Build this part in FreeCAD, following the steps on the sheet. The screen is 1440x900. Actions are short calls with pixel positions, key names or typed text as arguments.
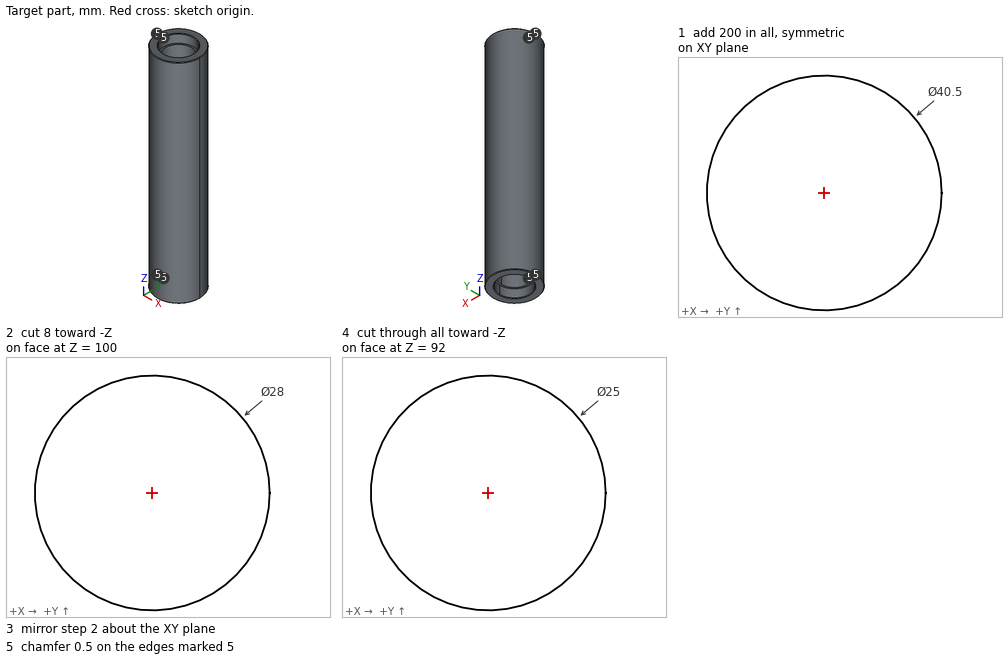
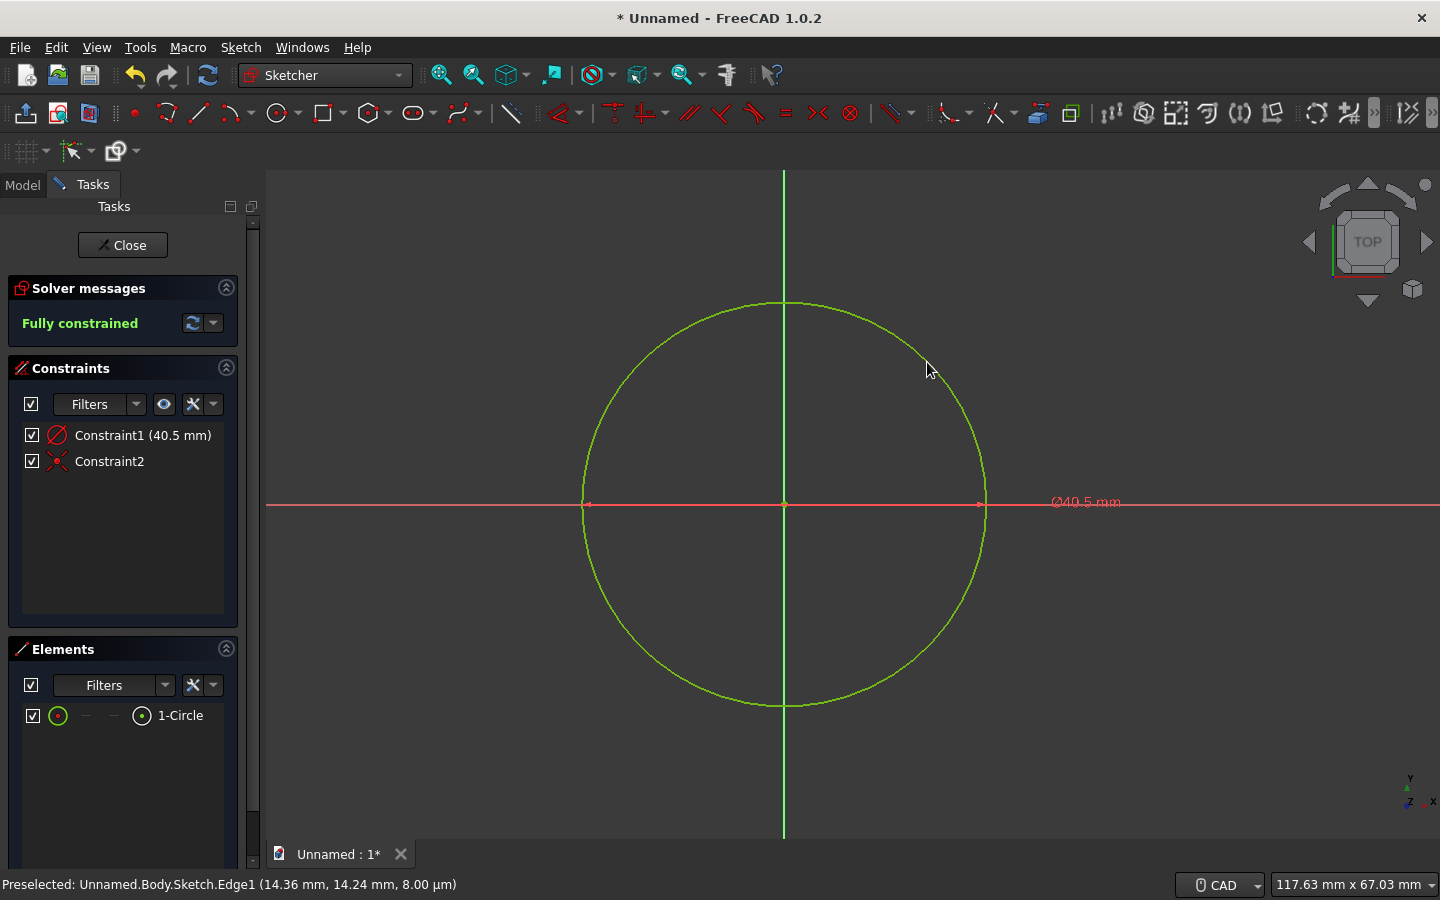
click(123, 245)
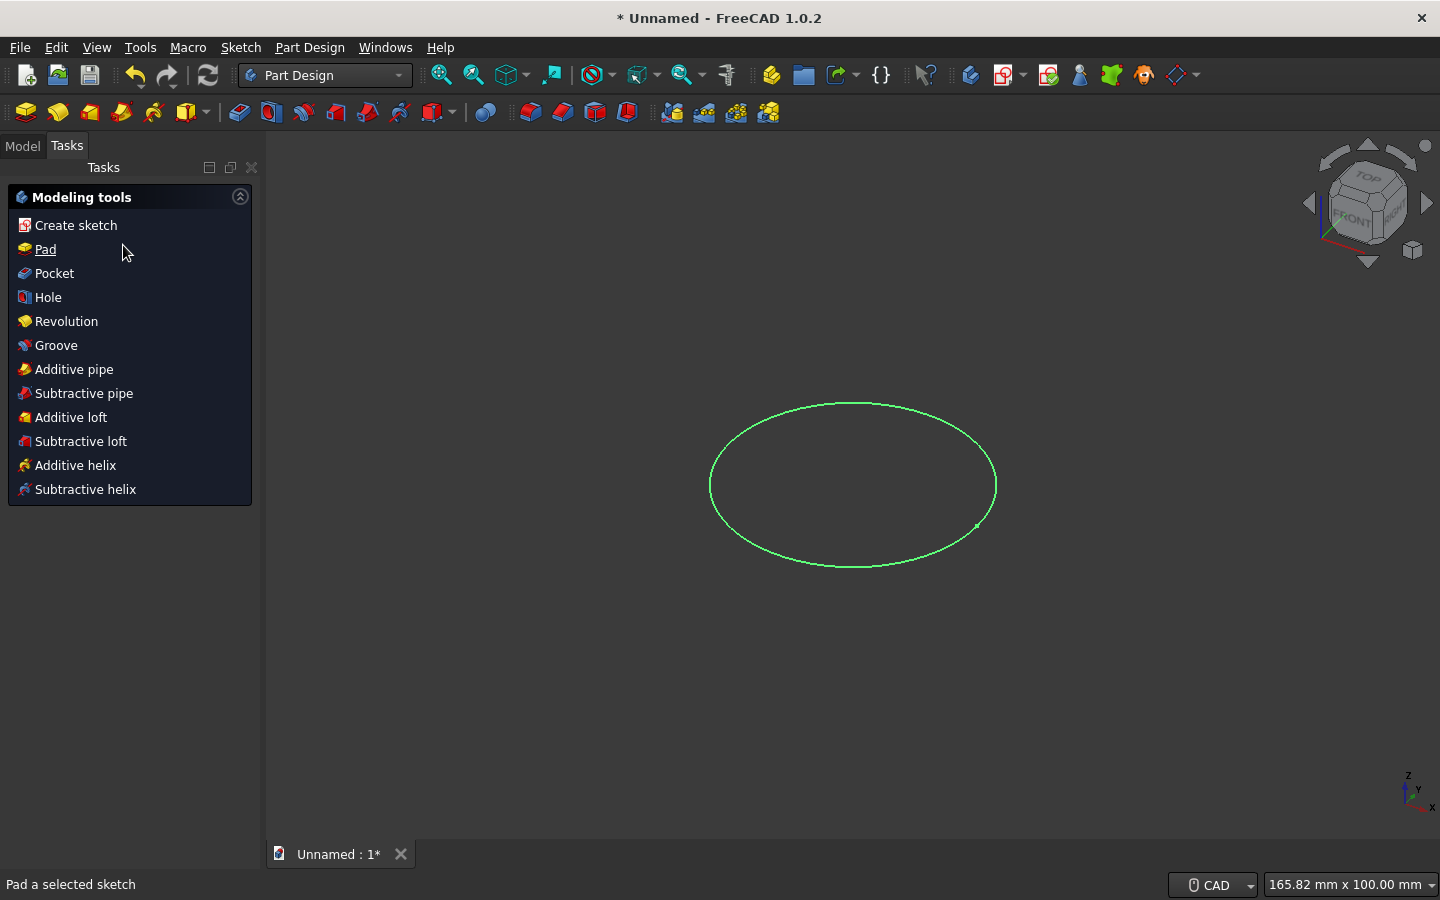
click(26, 112)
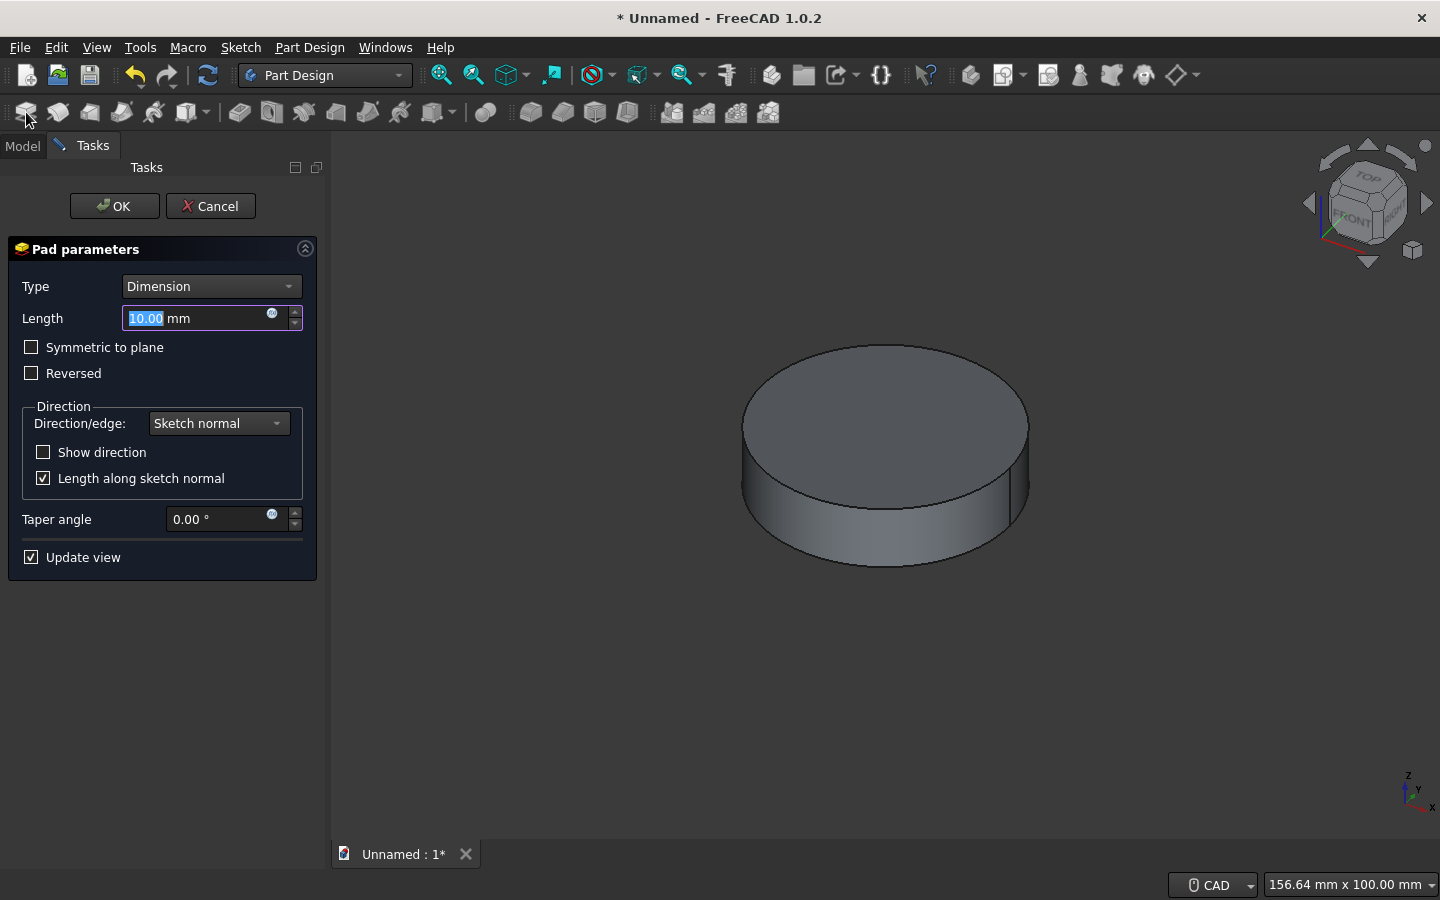
text(200)
key(Tab)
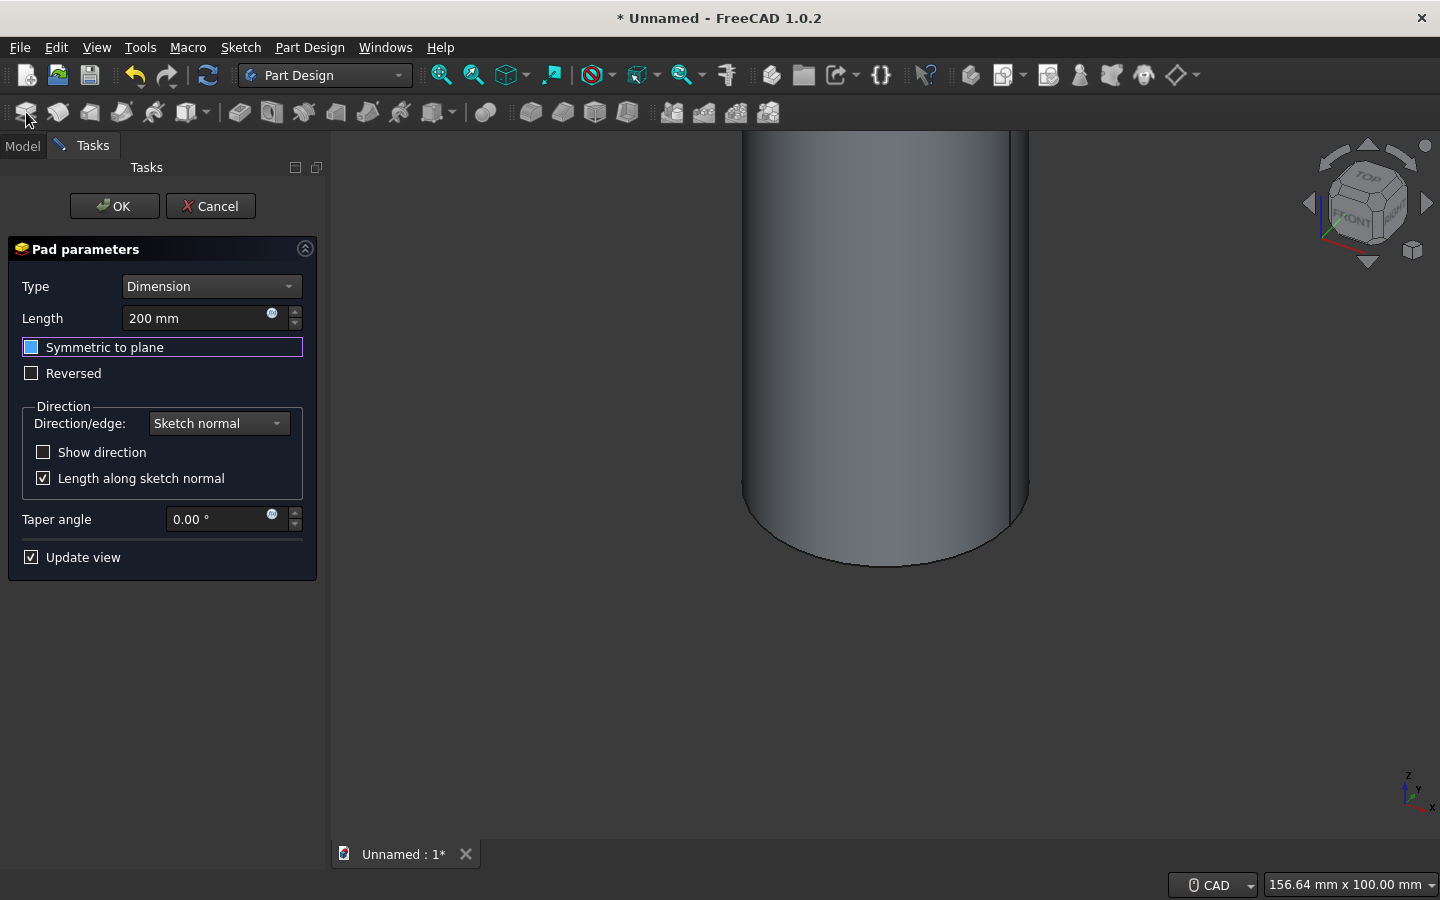
click(30, 347)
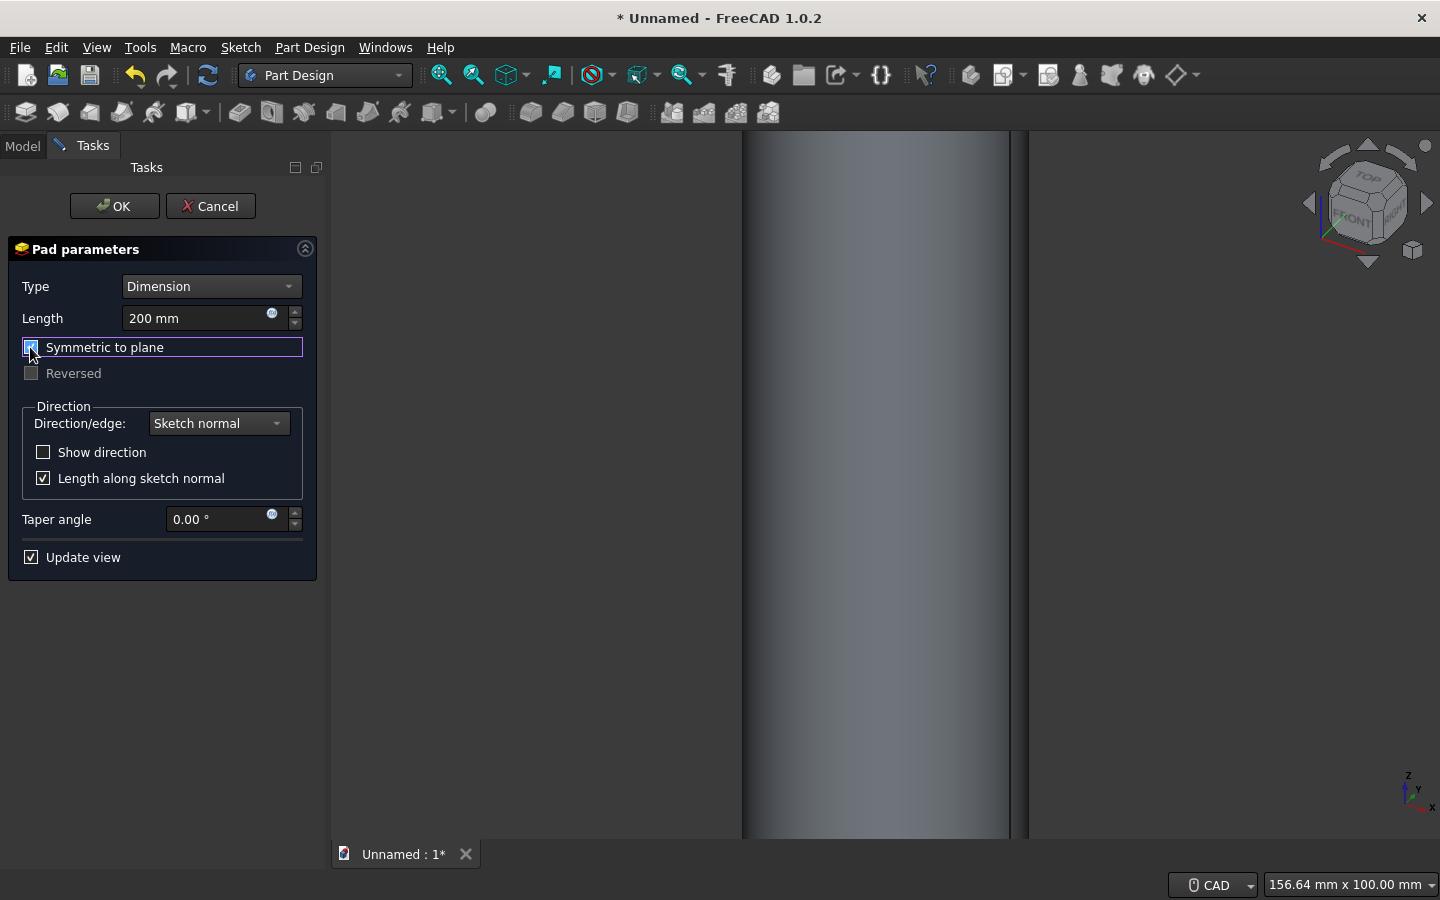
click(115, 206)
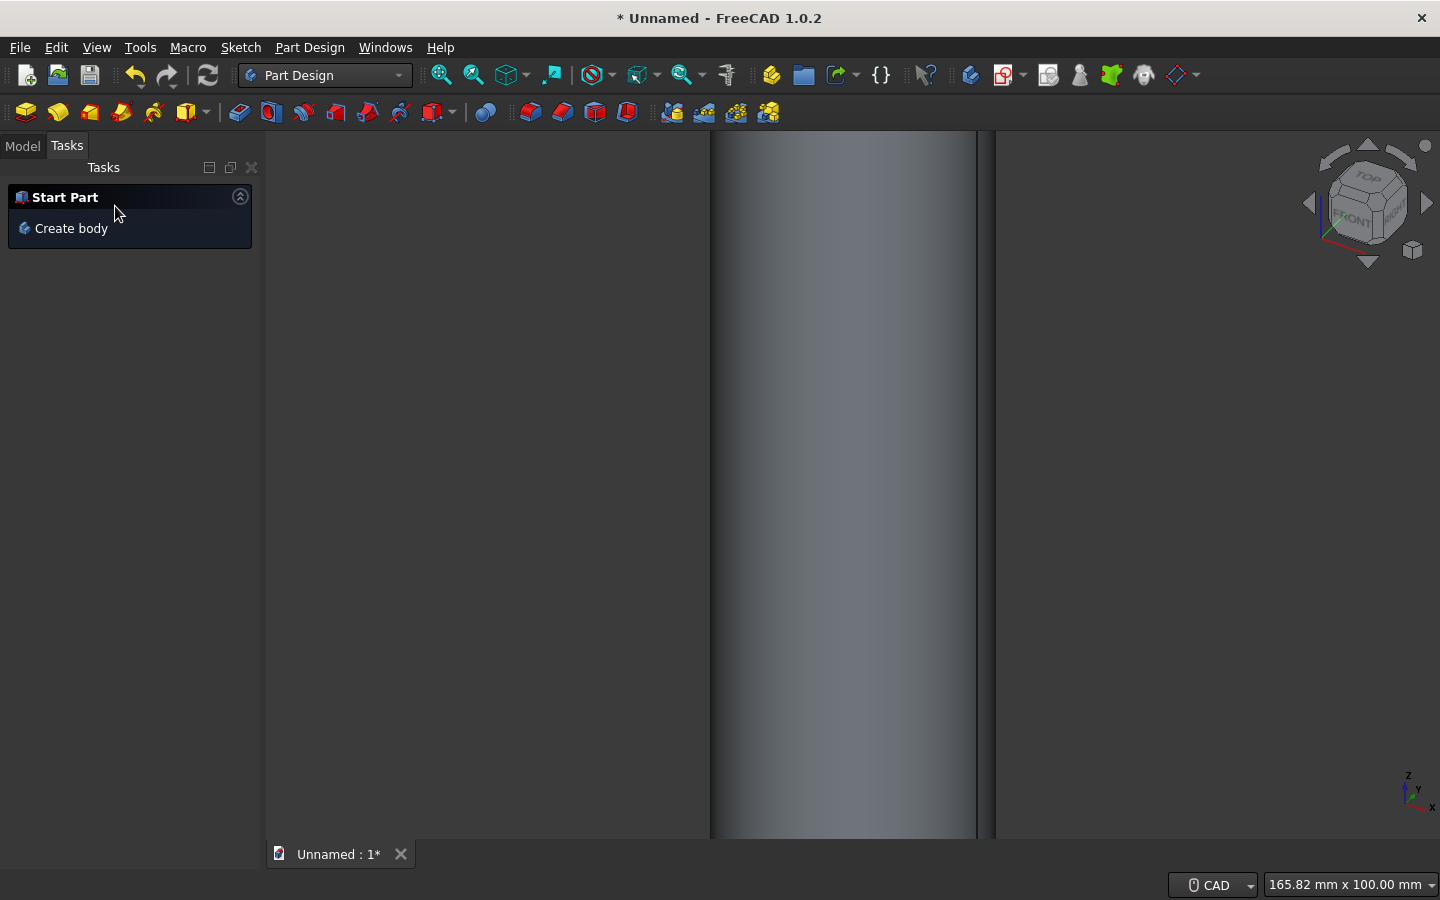
click(442, 76)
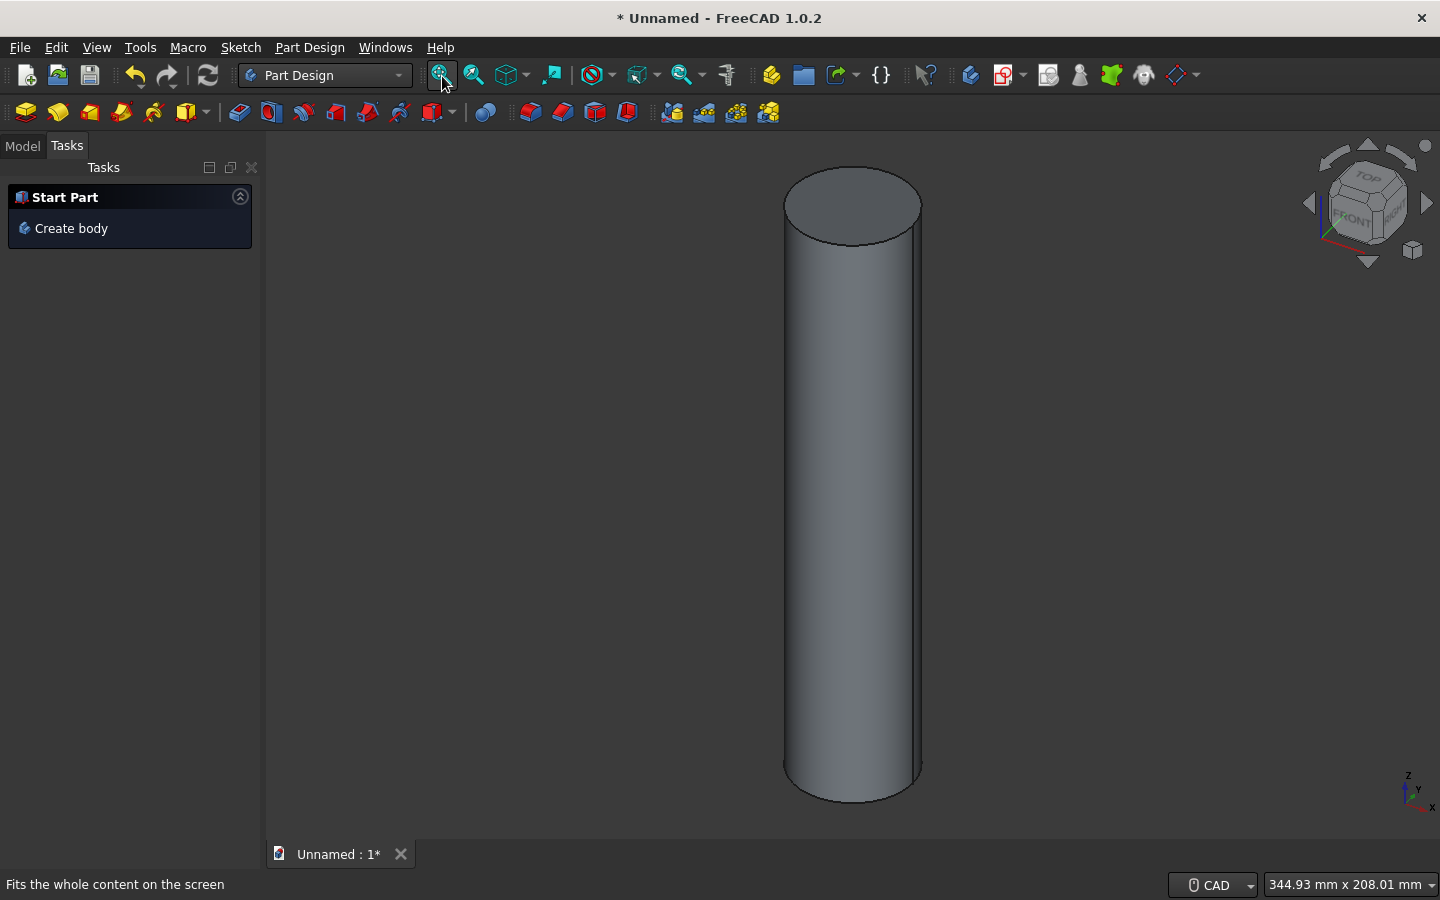
click(853, 205)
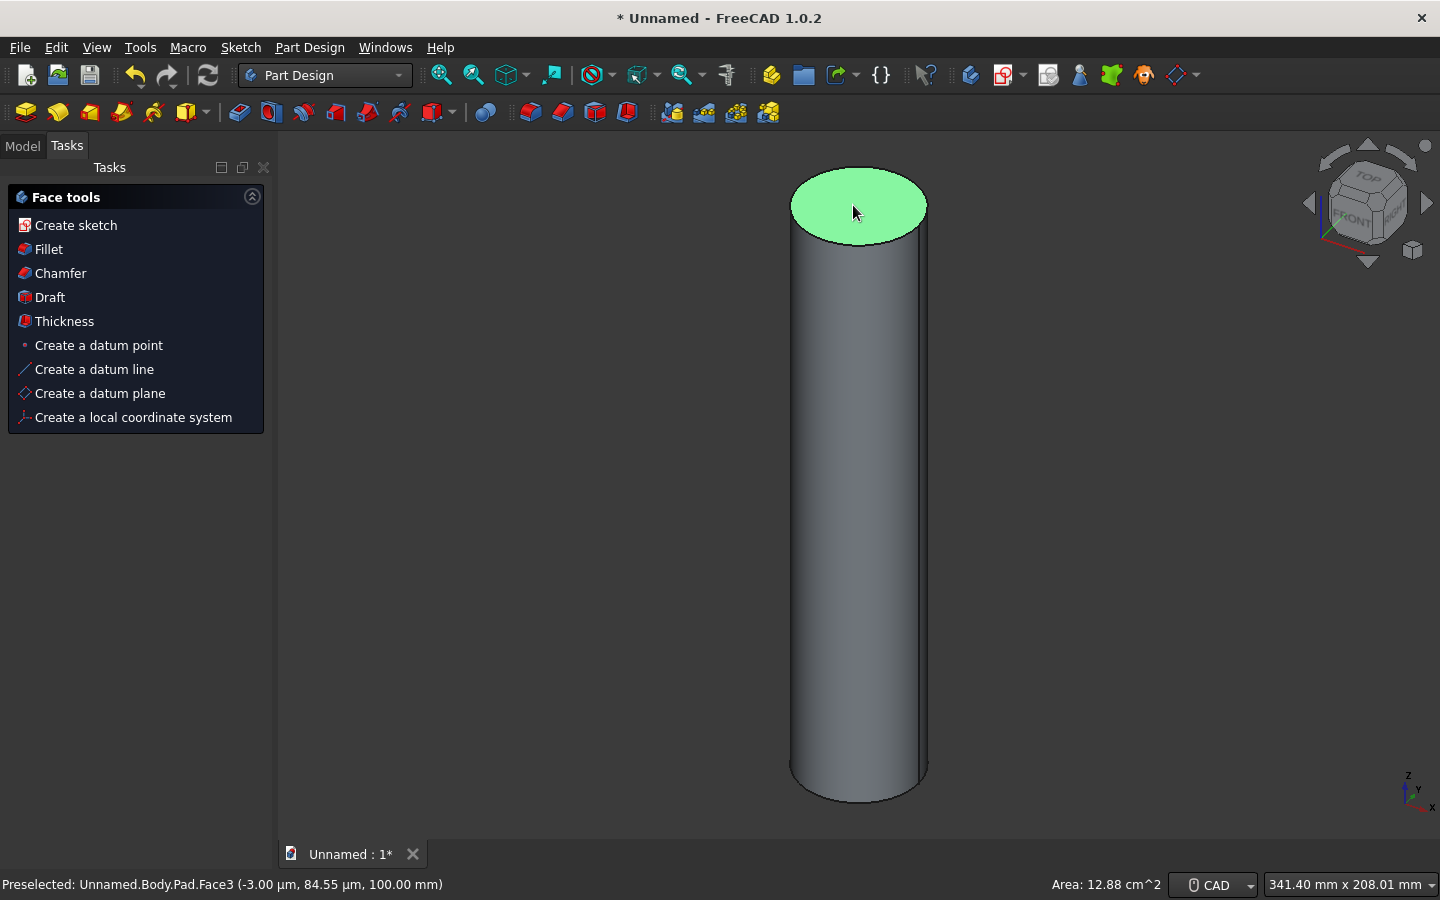
click(1004, 76)